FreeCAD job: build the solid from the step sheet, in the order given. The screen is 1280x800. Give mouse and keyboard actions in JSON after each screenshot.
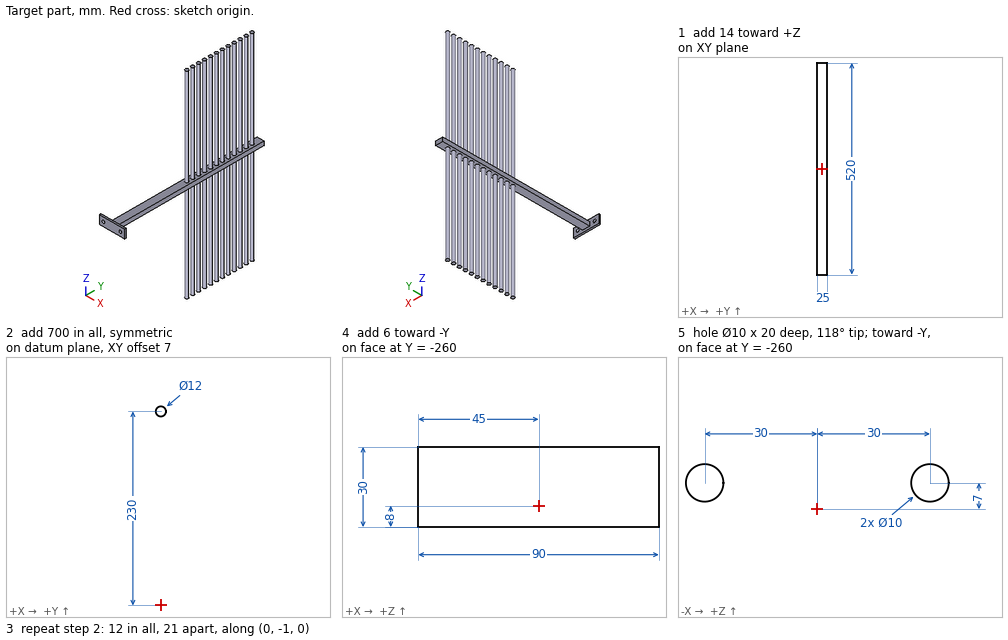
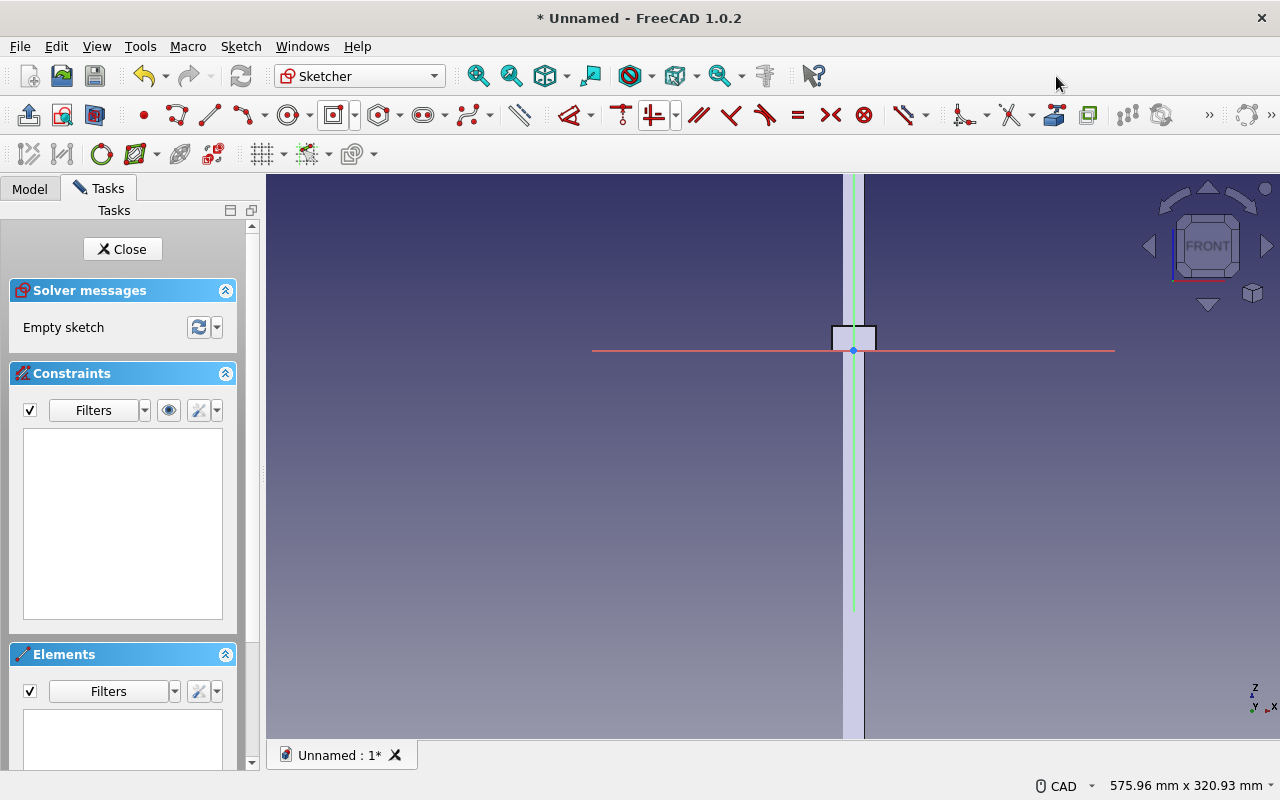
{"action": "scroll", "coordinate": [918, 288], "scroll_direction": "up", "scroll_amount": 6}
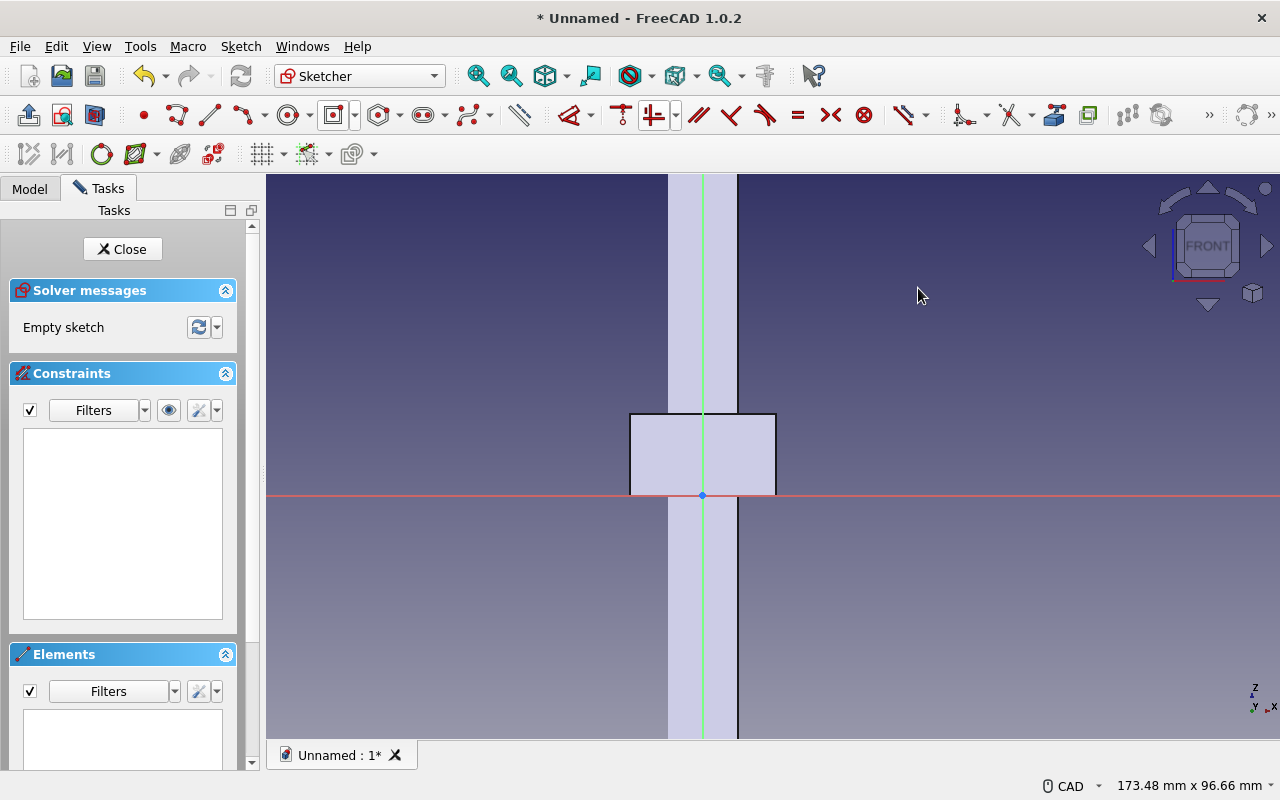
{"action": "left_click", "coordinate": [354, 116]}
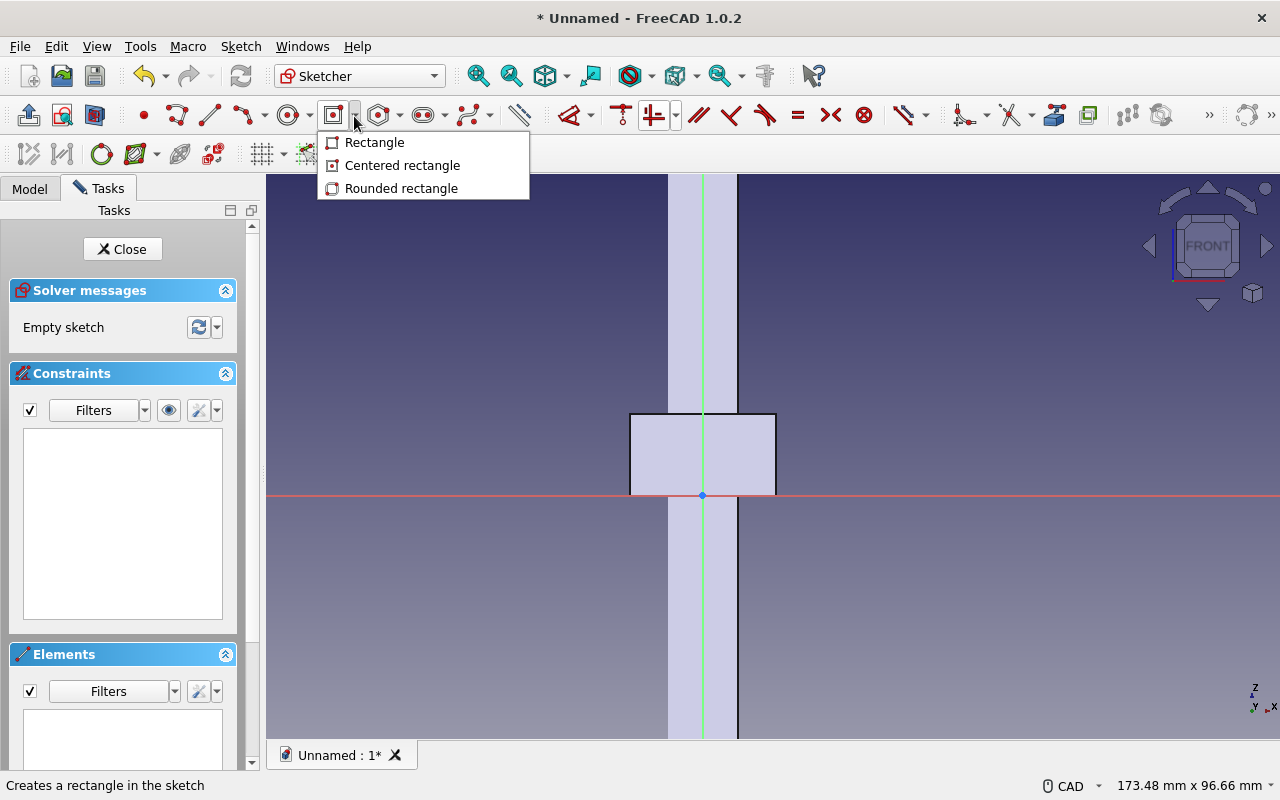
{"action": "left_click", "coordinate": [424, 142]}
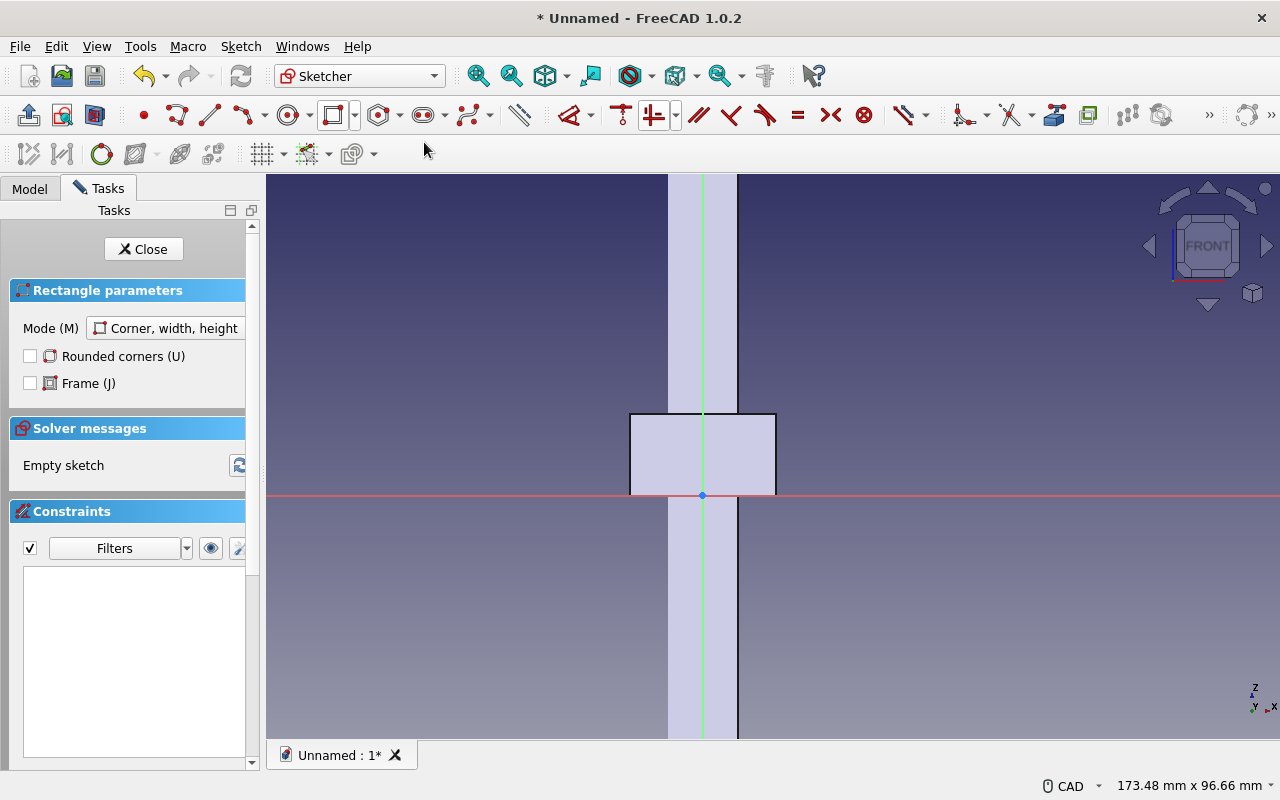
{"action": "left_click", "coordinate": [440, 367]}
{"action": "left_click", "coordinate": [966, 543]}
{"action": "key", "text": "Escape"}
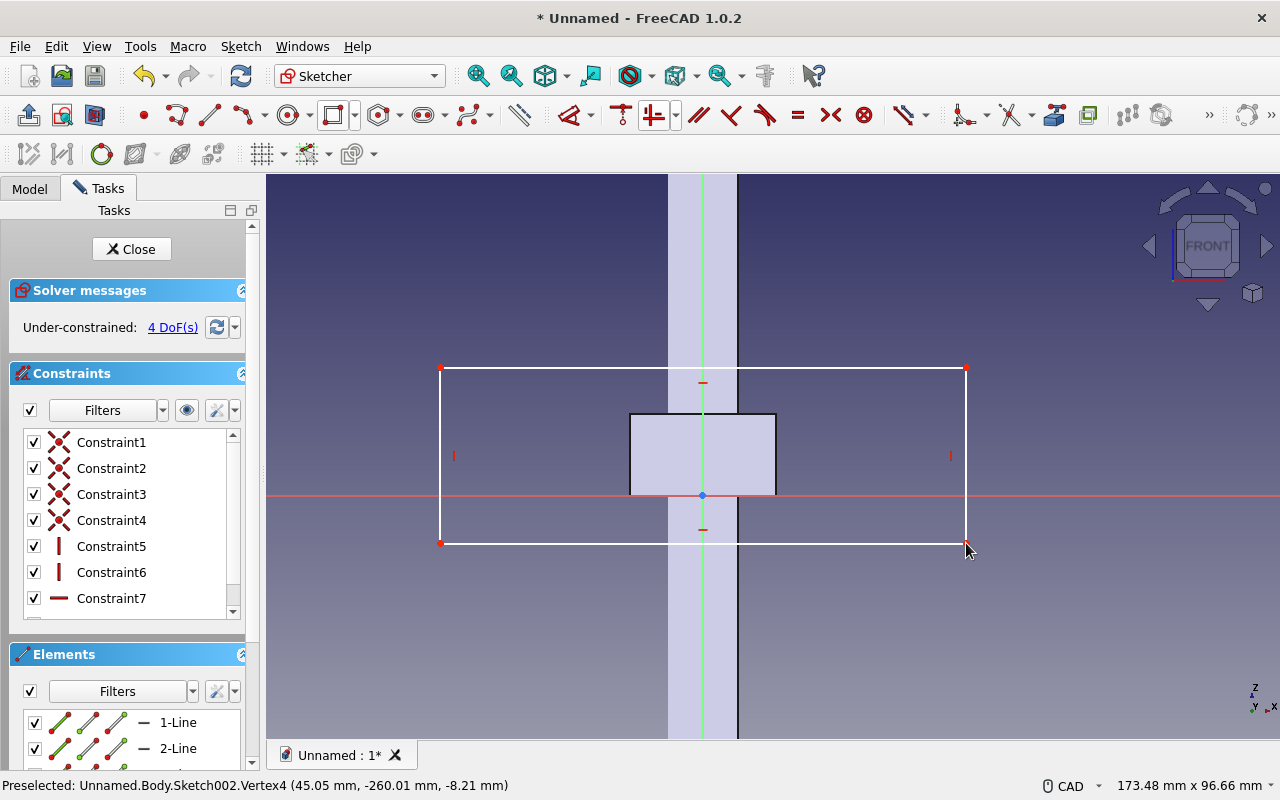
{"action": "left_click", "coordinate": [568, 116]}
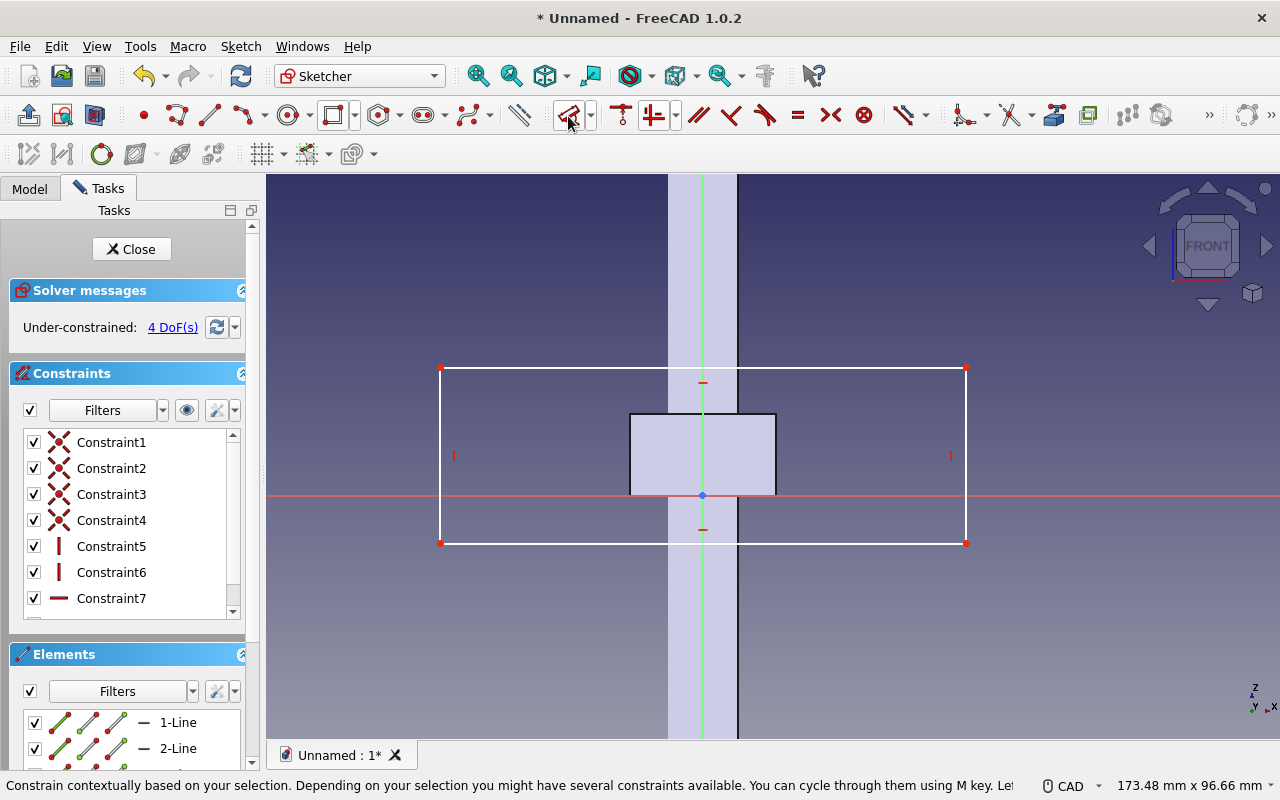
{"action": "left_click", "coordinate": [440, 421]}
{"action": "left_click", "coordinate": [406, 456]}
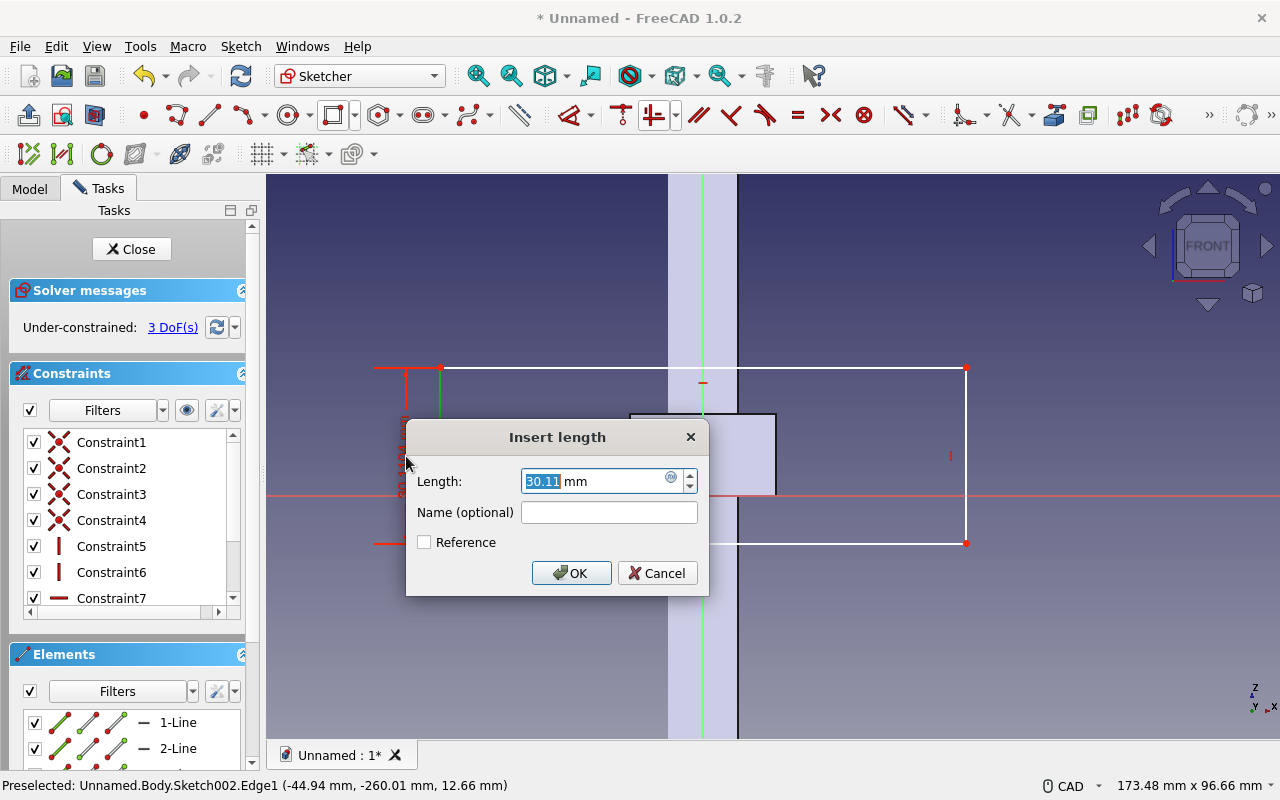
{"action": "type", "text": "30"}
{"action": "key", "text": "Return"}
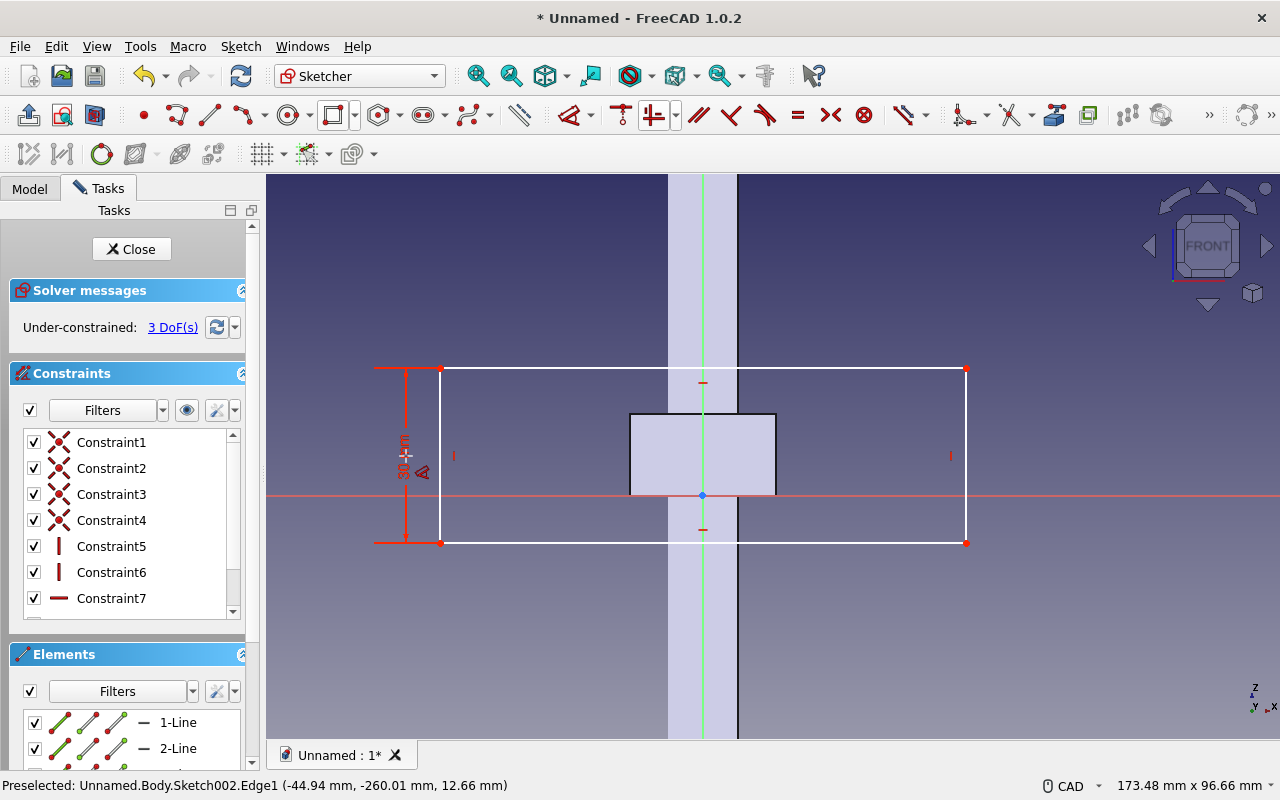
{"action": "left_click", "coordinate": [598, 543]}
{"action": "left_click", "coordinate": [582, 577]}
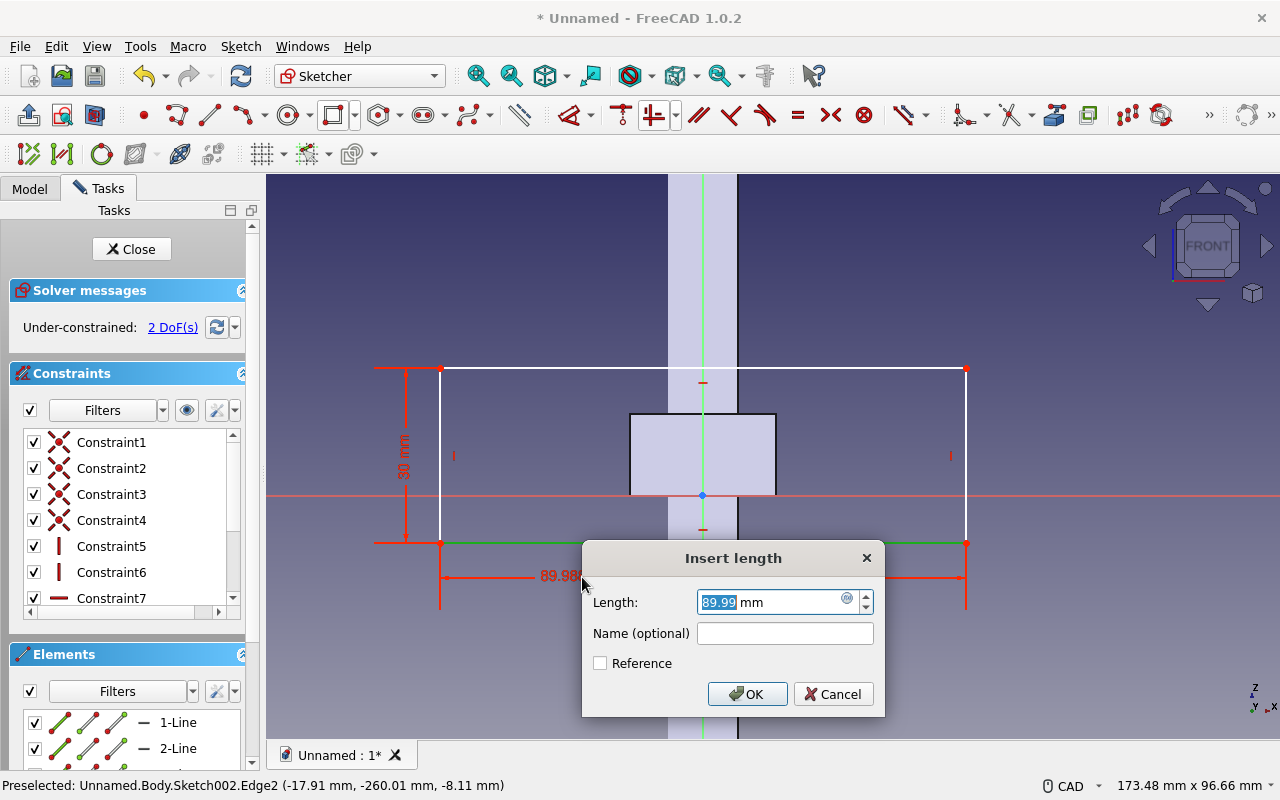
{"action": "type", "text": "90"}
{"action": "key", "text": "Return"}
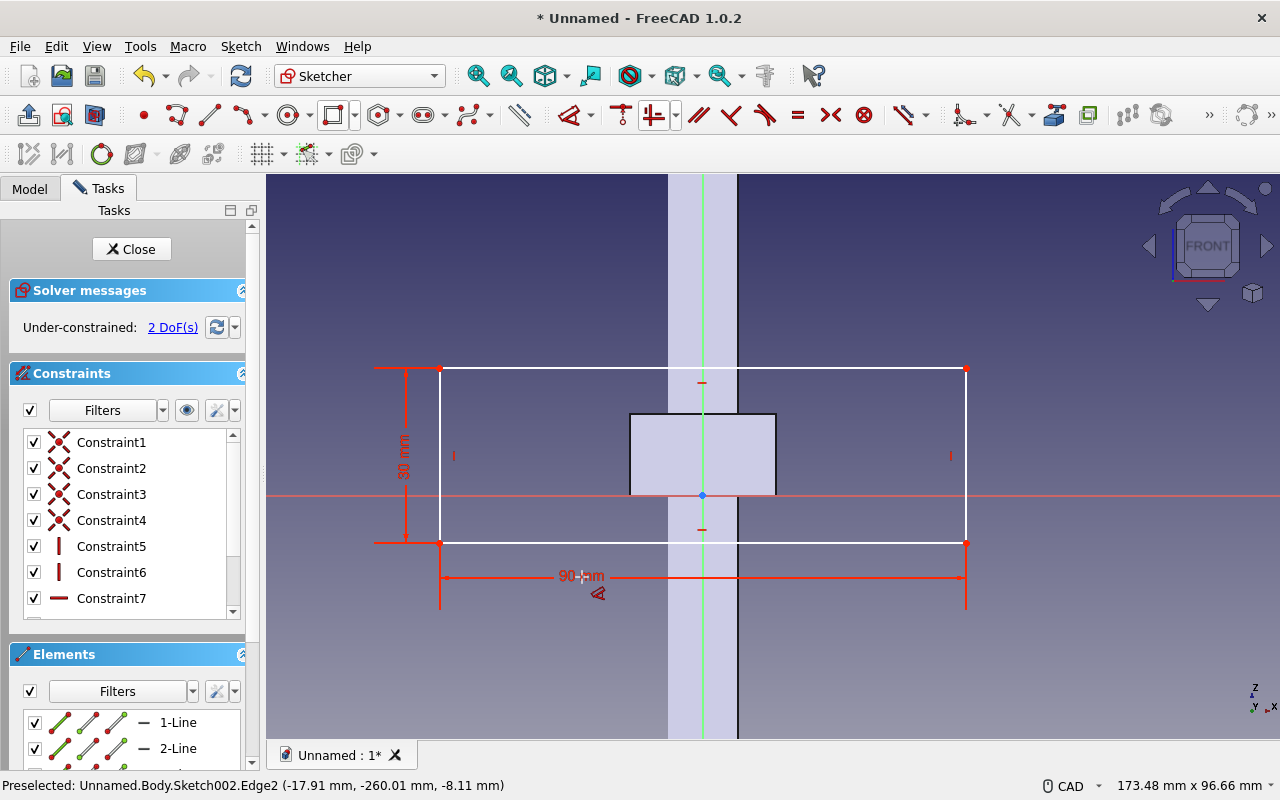
{"action": "left_click", "coordinate": [440, 543]}
{"action": "left_click", "coordinate": [406, 520]}